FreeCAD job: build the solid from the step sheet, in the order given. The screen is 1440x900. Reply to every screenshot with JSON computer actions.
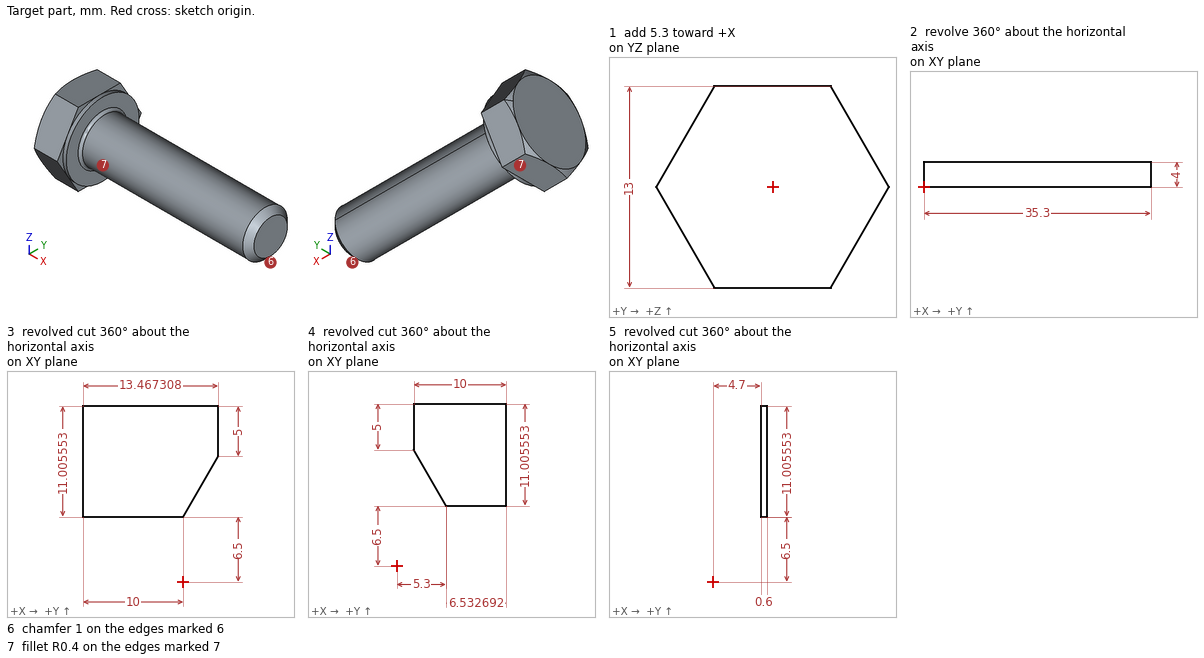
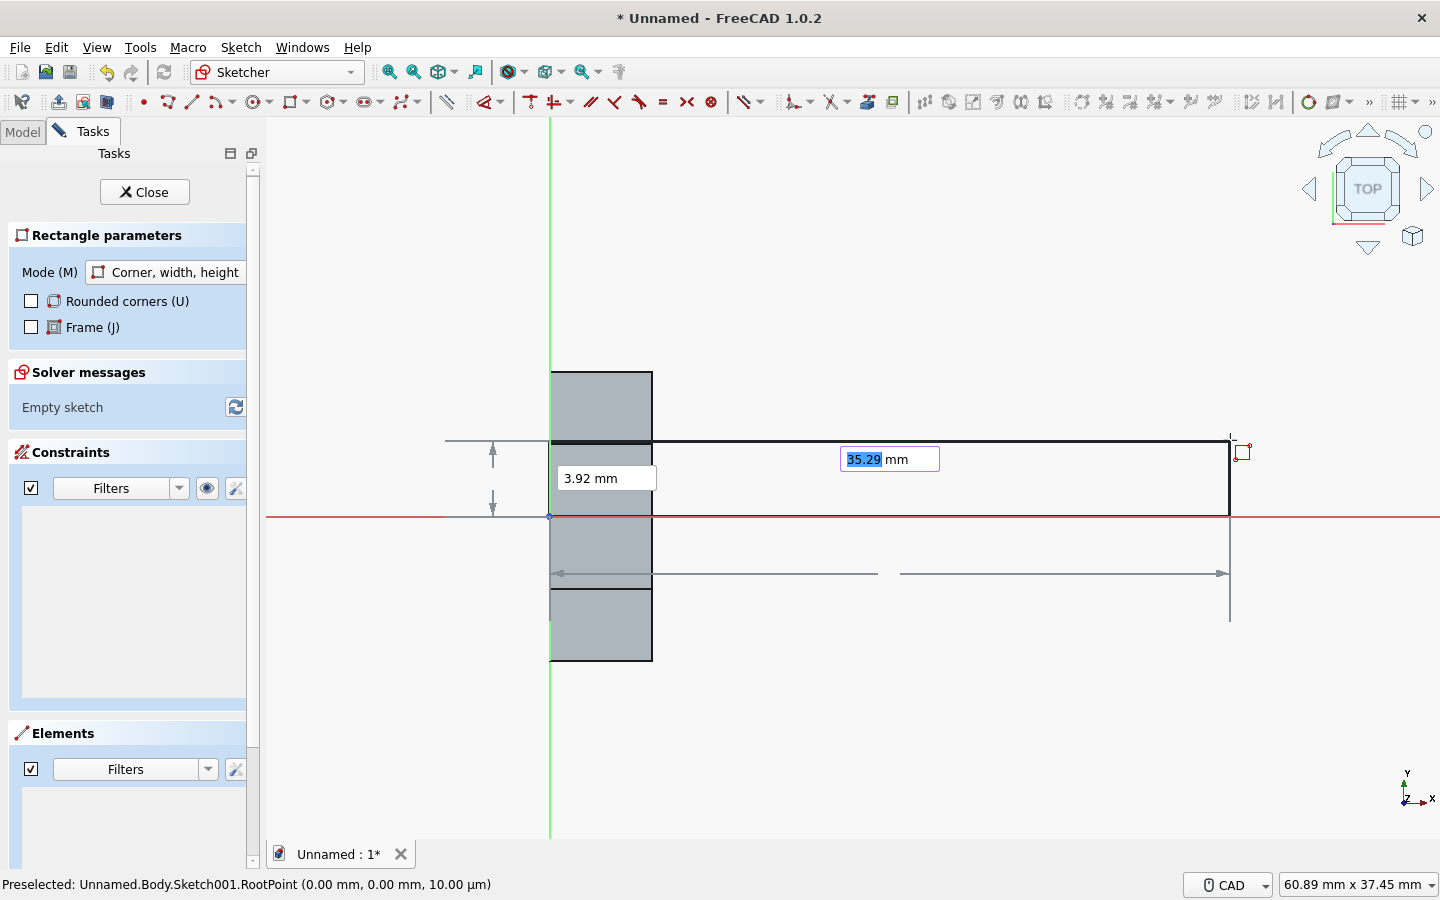
{"action": "type", "text": "35.3"}
{"action": "key", "text": "Tab"}
{"action": "type", "text": "4"}
{"action": "key", "text": "Return"}
{"action": "key", "text": "Escape"}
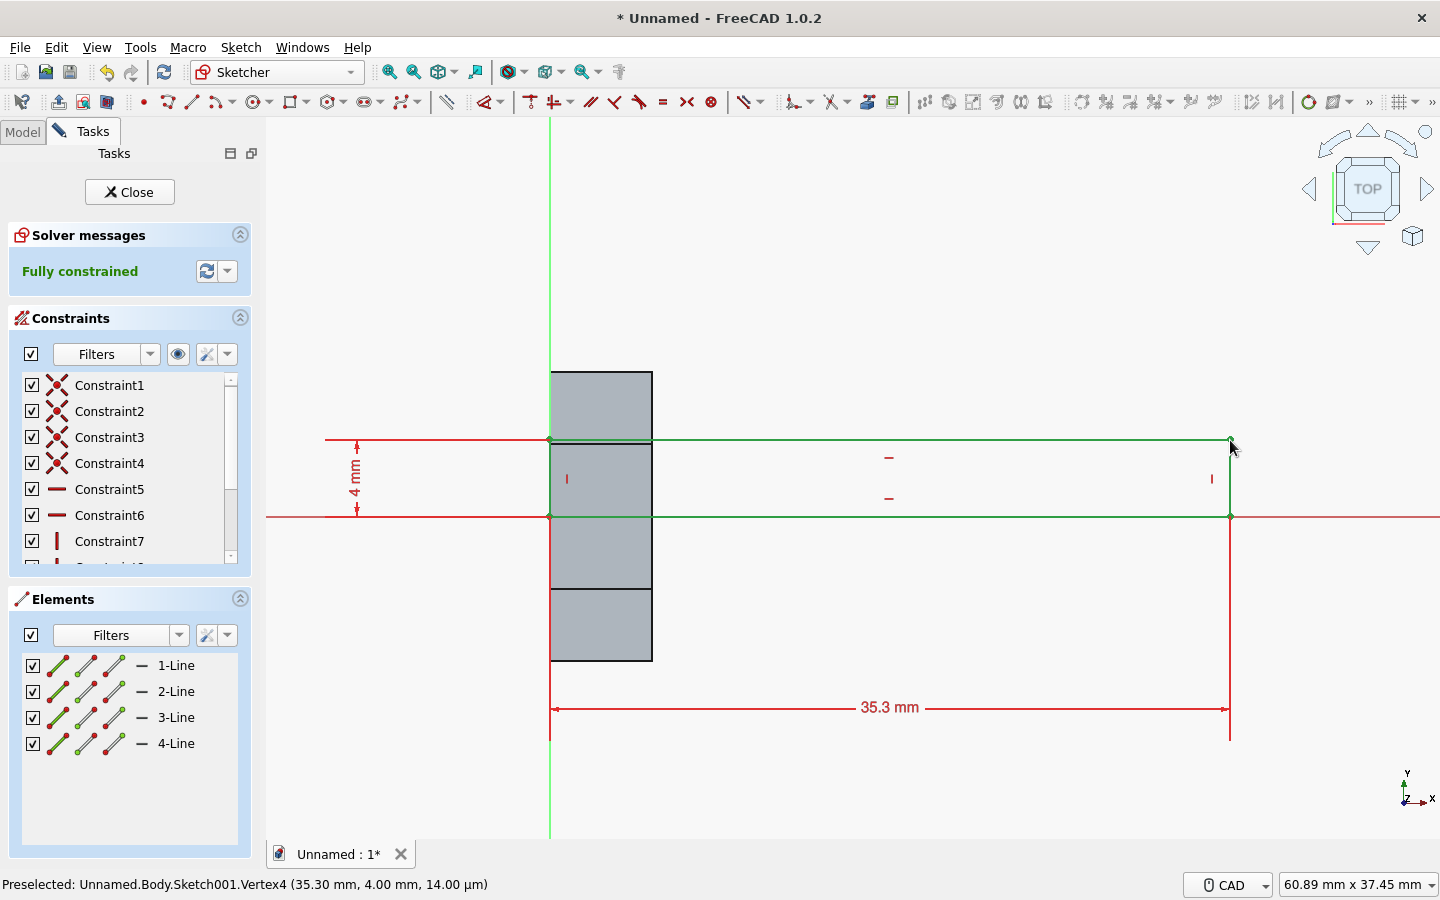
{"action": "left_click", "coordinate": [130, 192]}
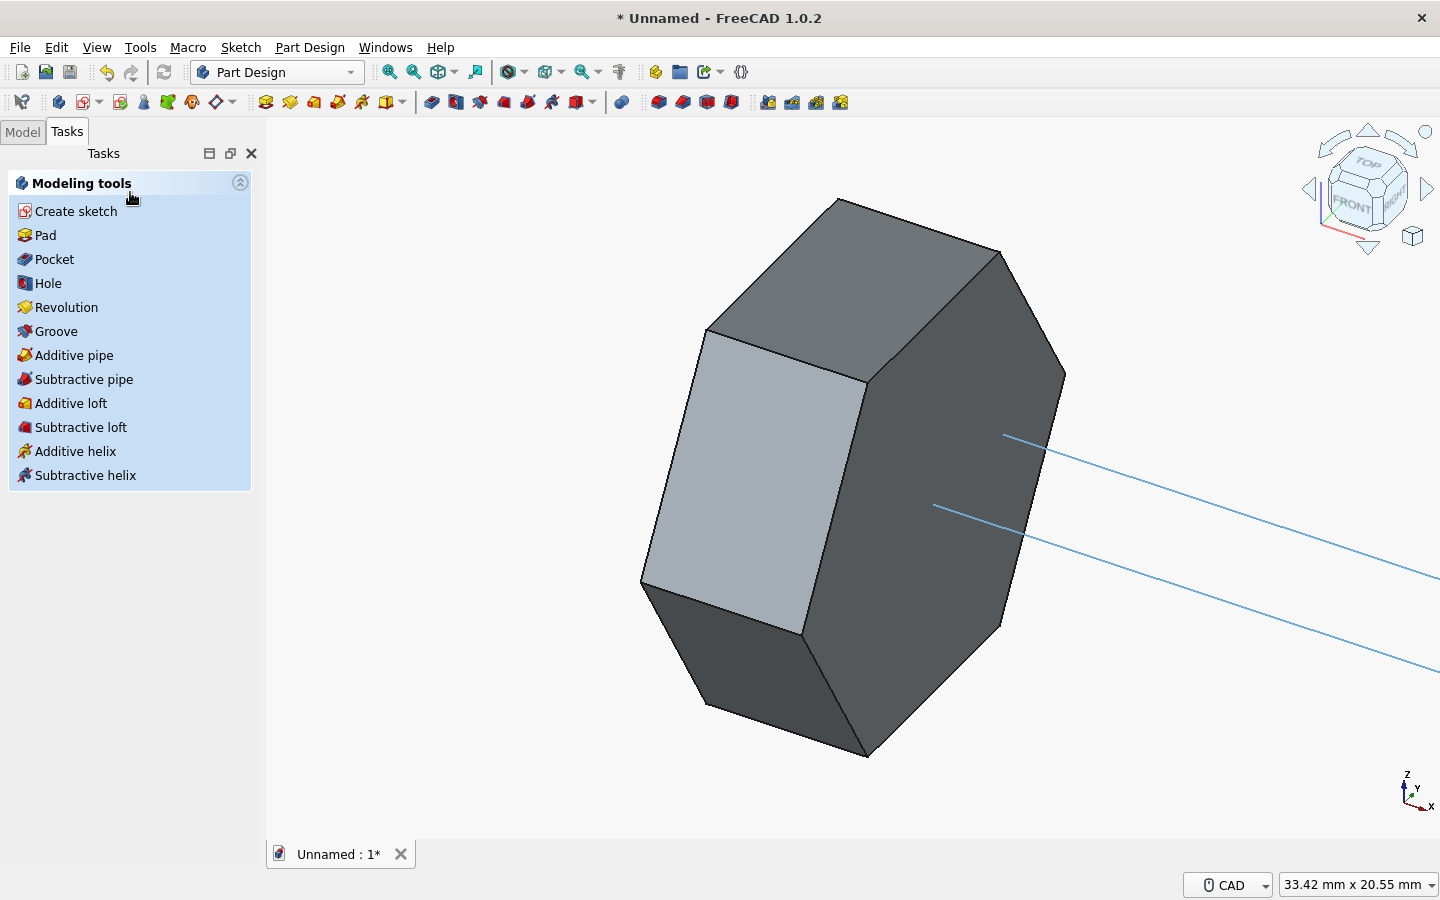
{"action": "left_click", "coordinate": [290, 102]}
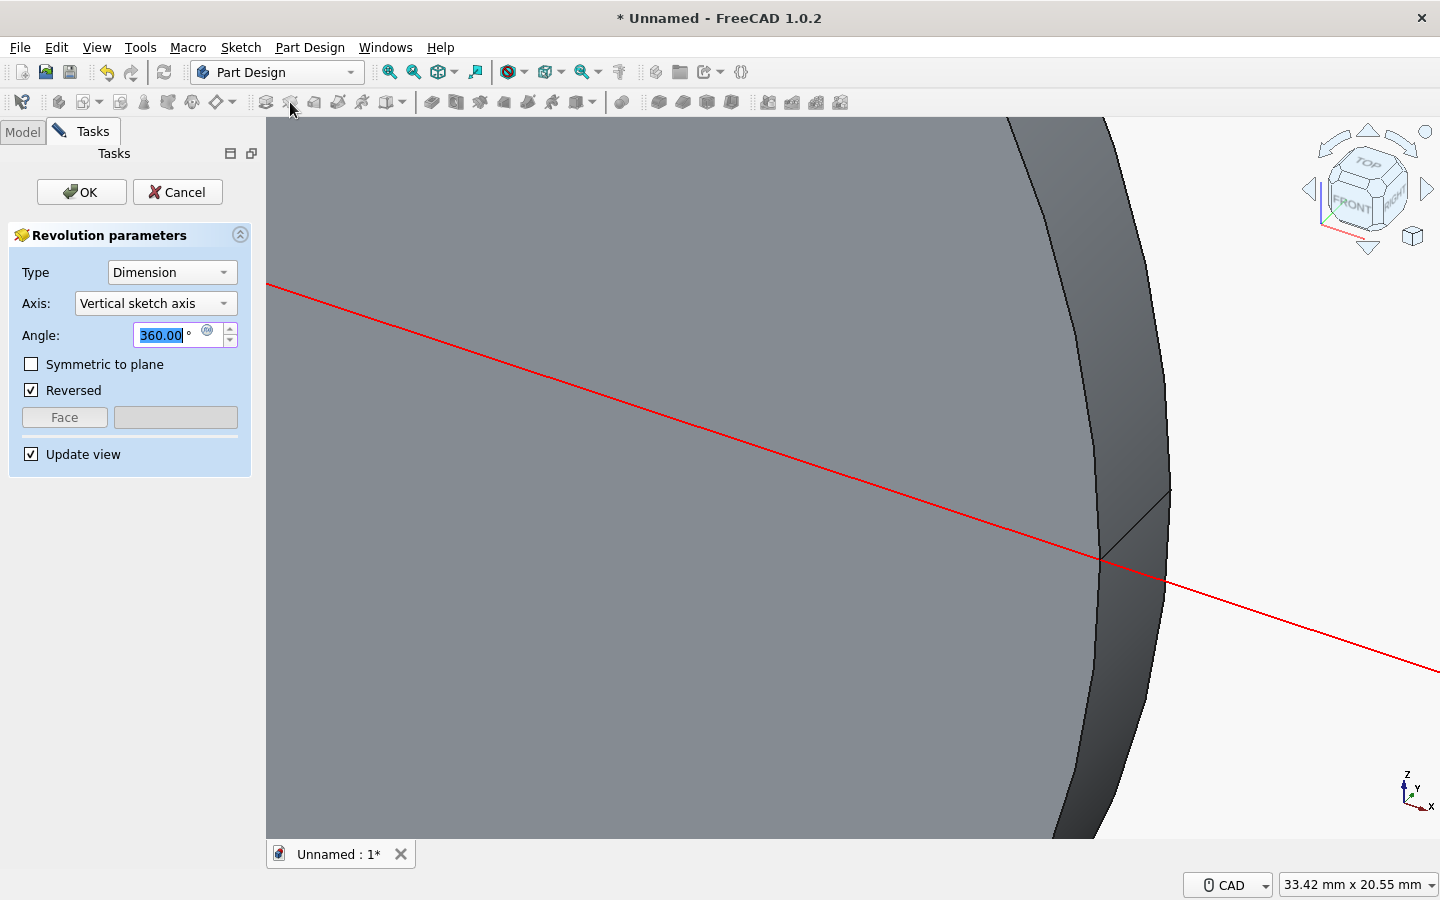
{"action": "left_click", "coordinate": [156, 304]}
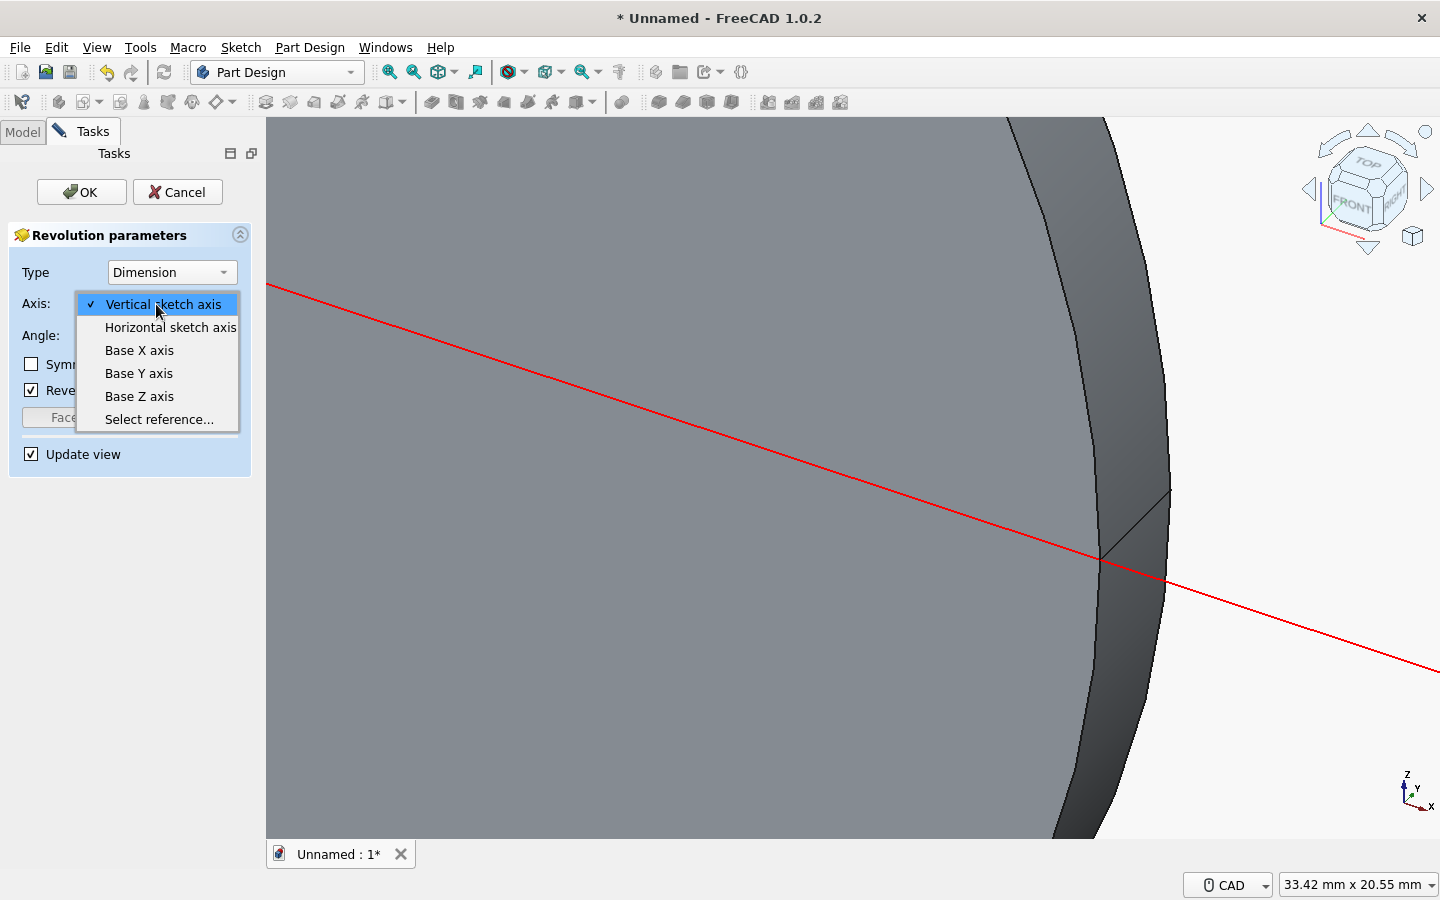
{"action": "left_click", "coordinate": [156, 328]}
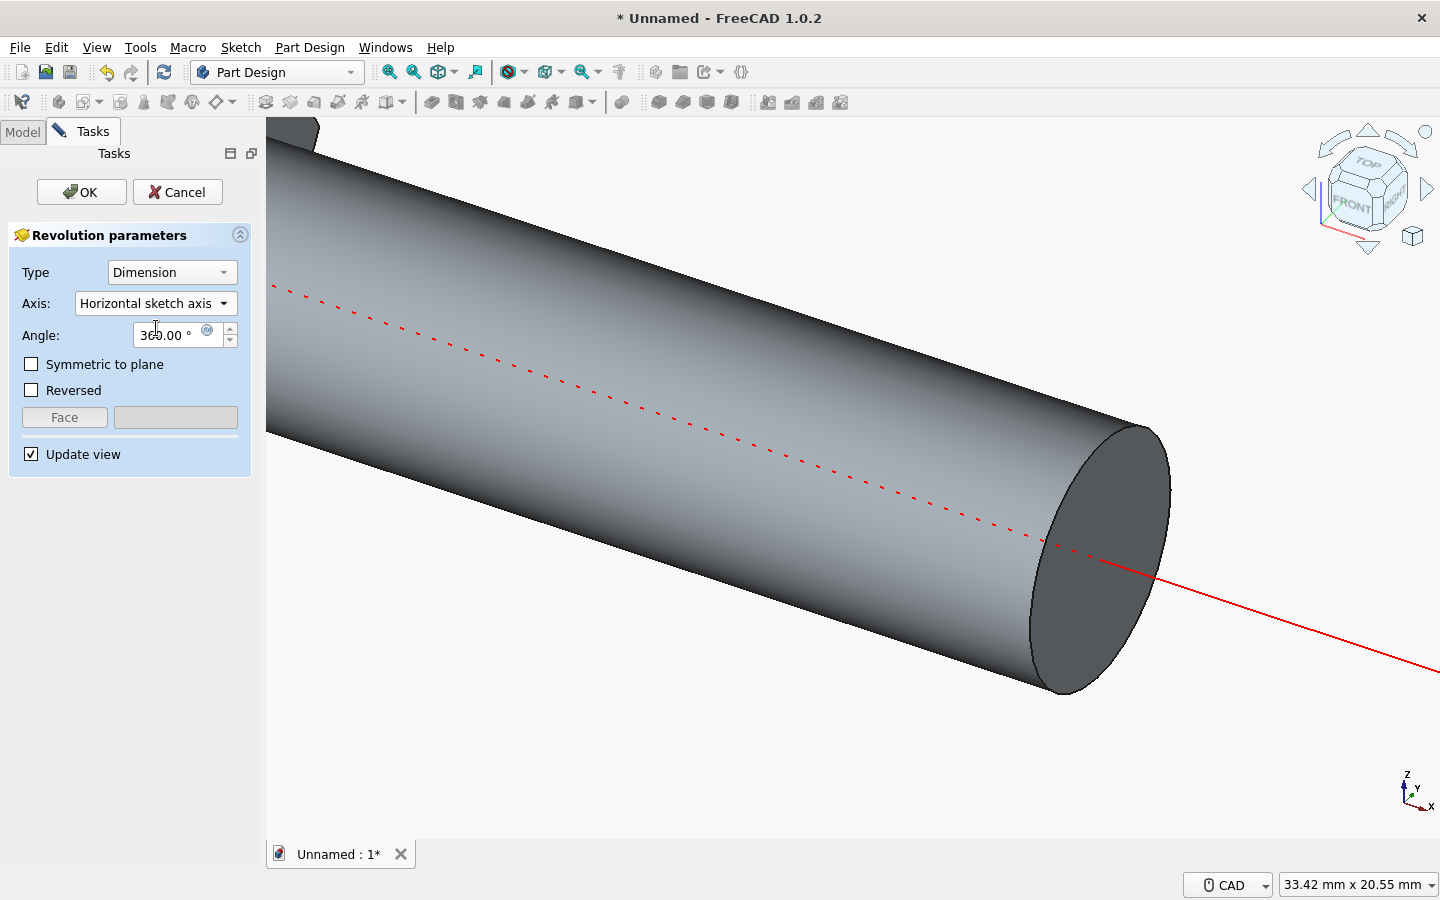
{"action": "left_click", "coordinate": [82, 192]}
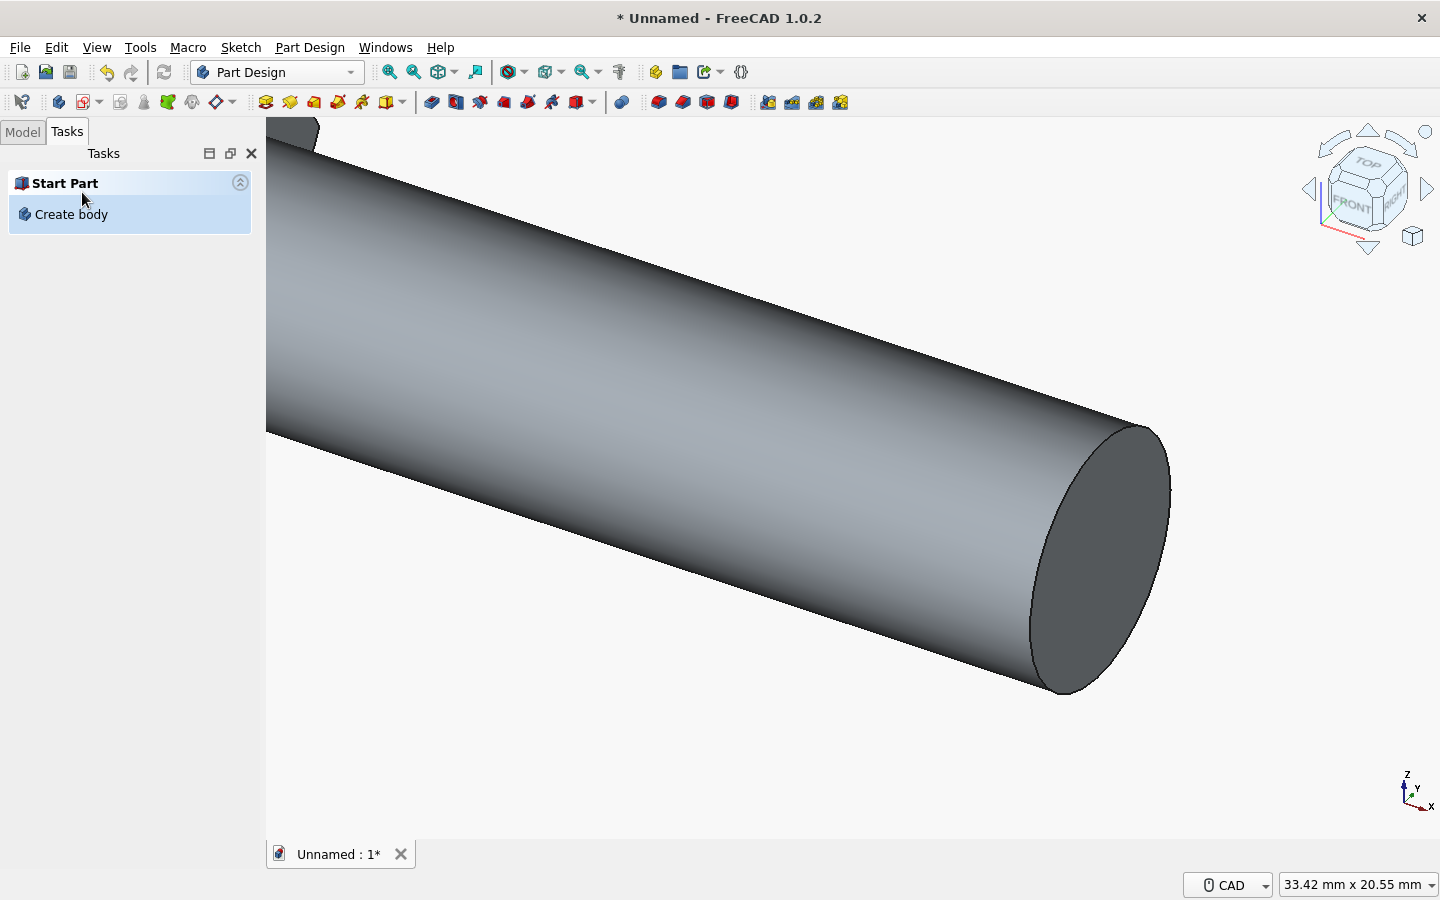
{"action": "key", "text": "v f"}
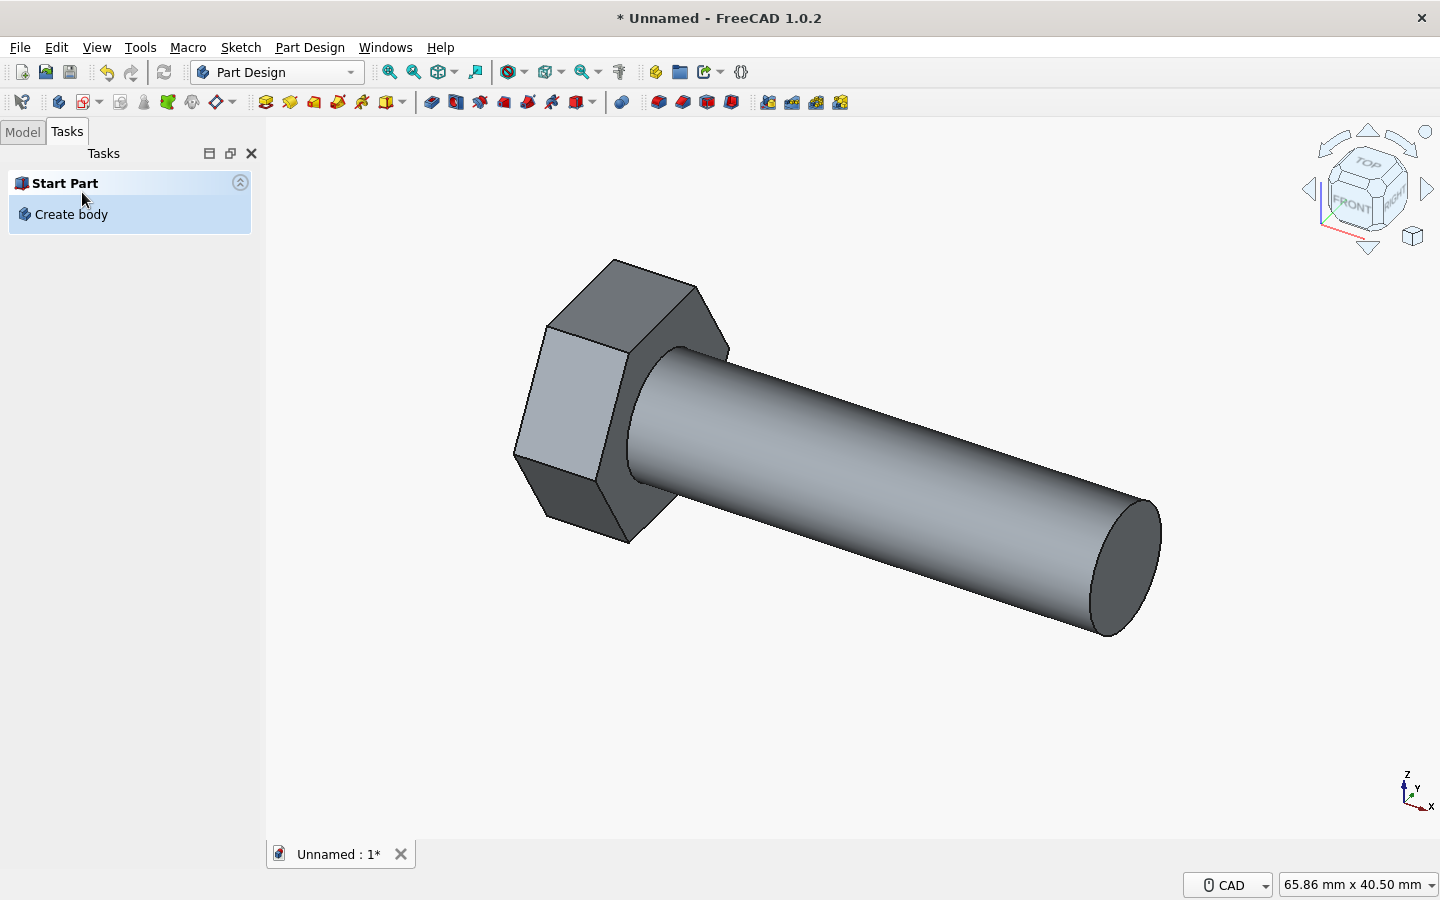
{"action": "left_click", "coordinate": [84, 102]}